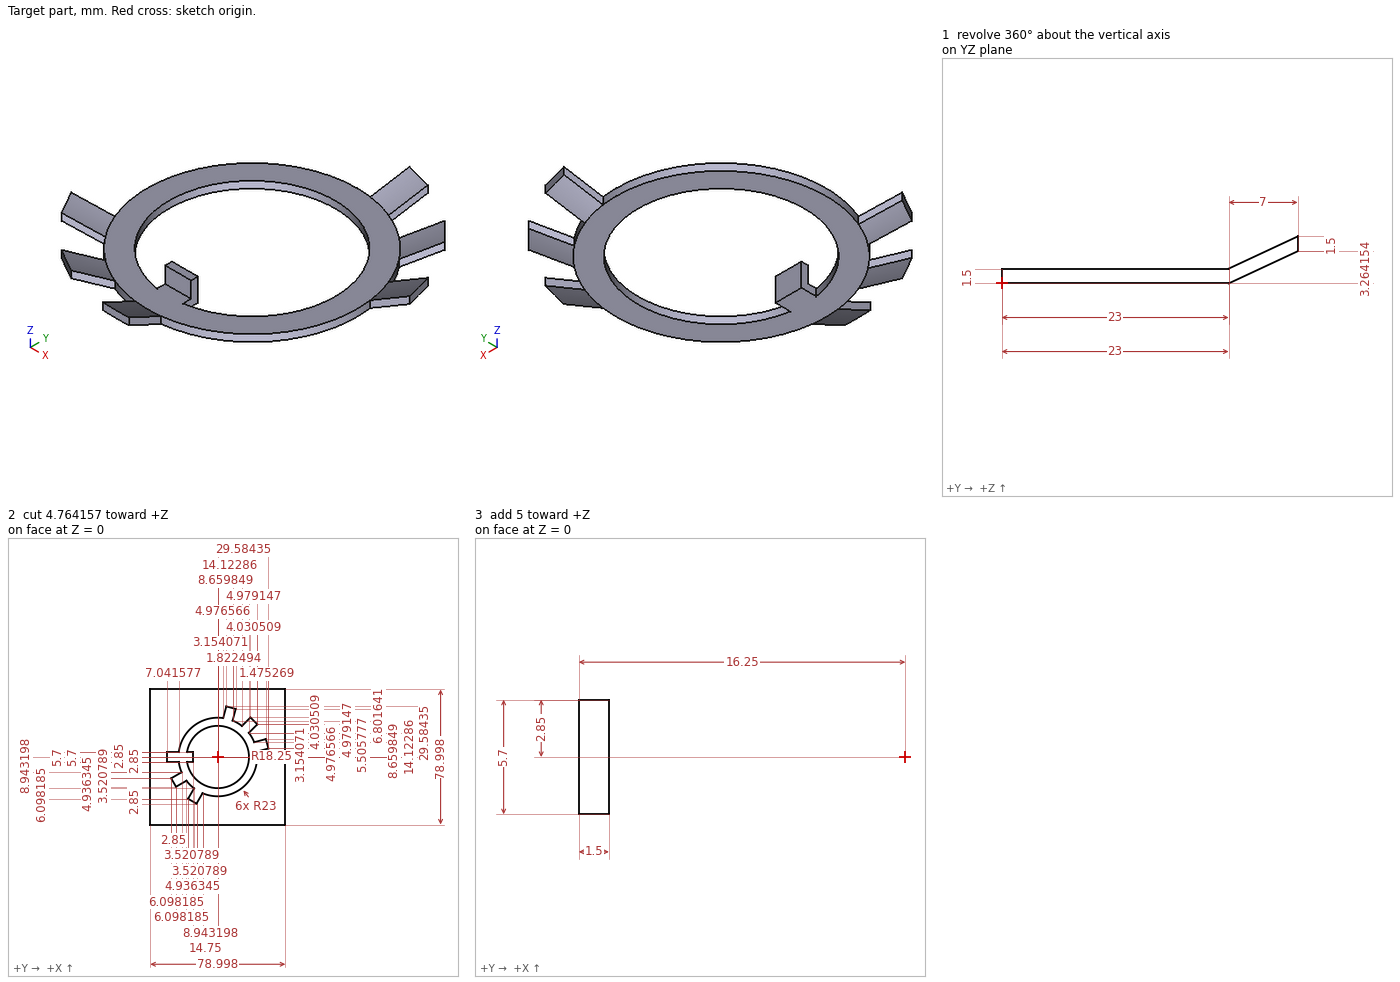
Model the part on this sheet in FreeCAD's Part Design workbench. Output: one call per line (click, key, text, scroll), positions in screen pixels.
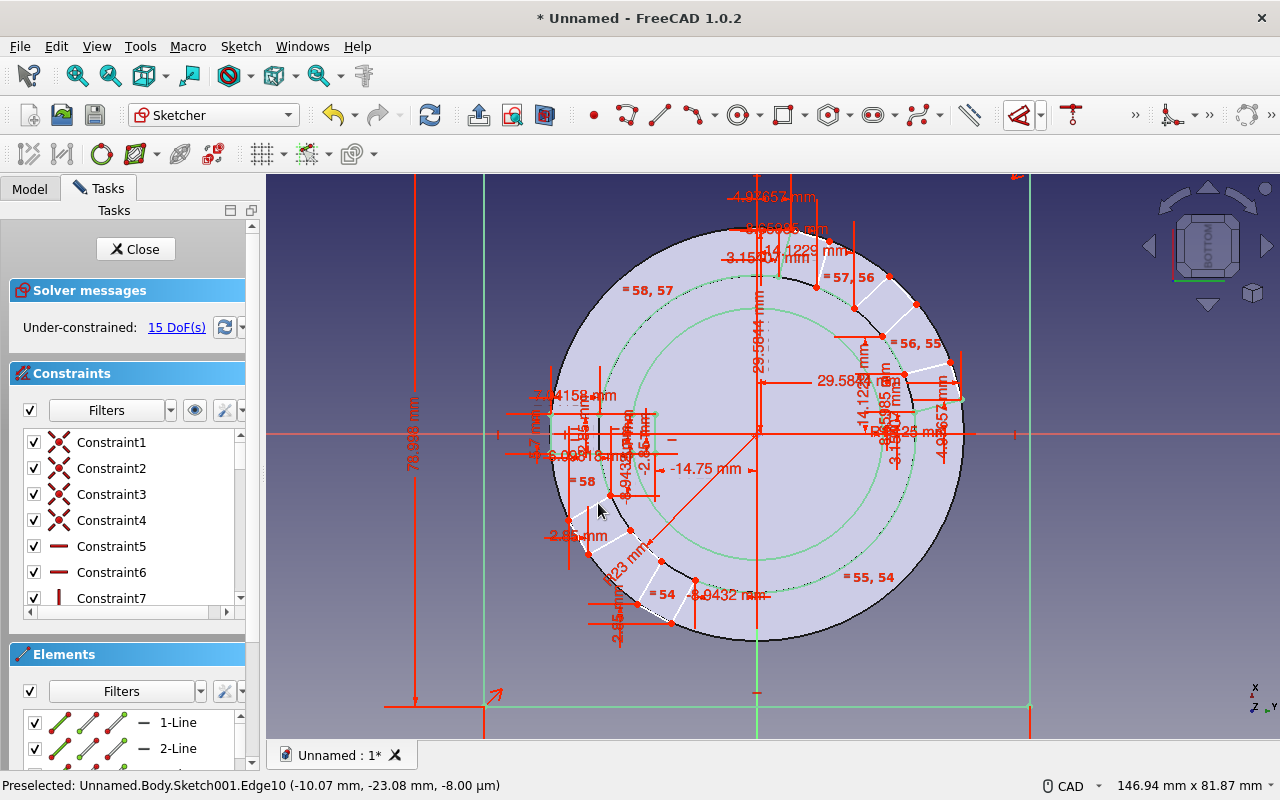
scroll(598, 503, up, 3)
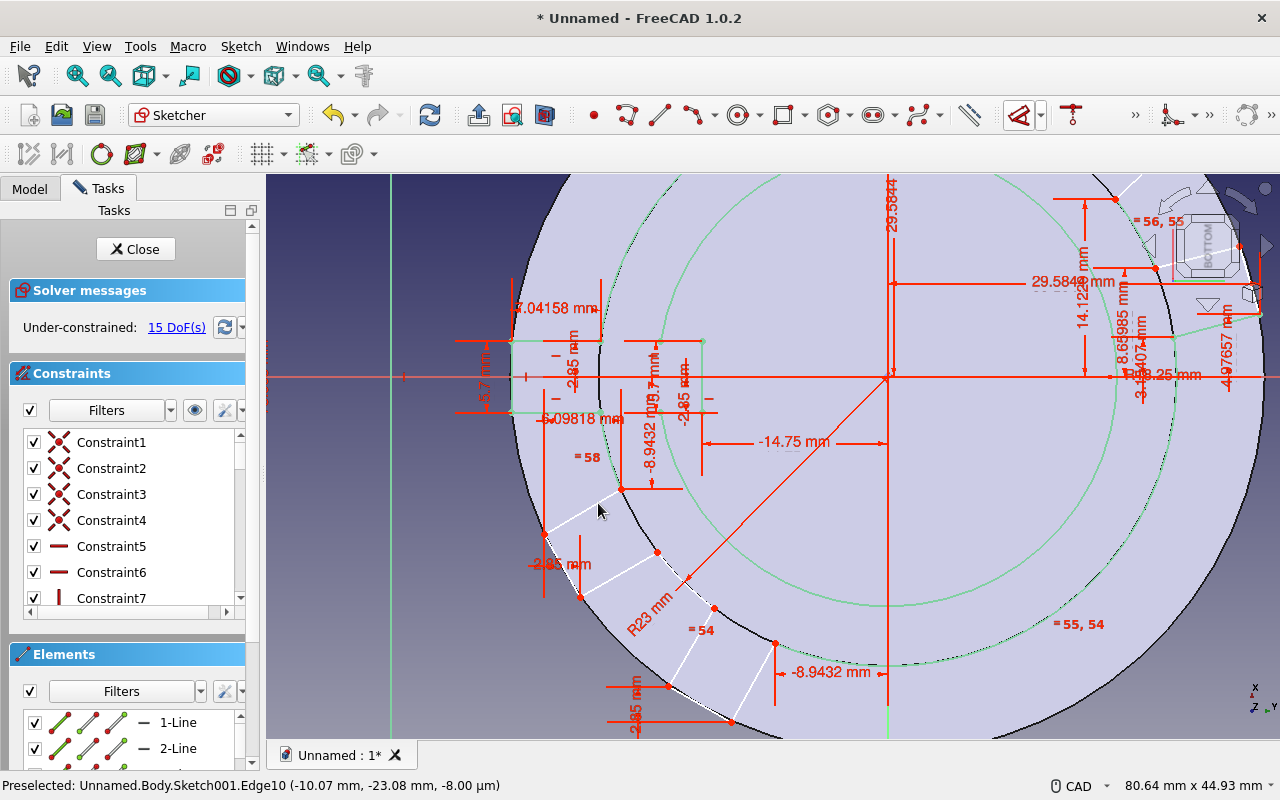
click(598, 503)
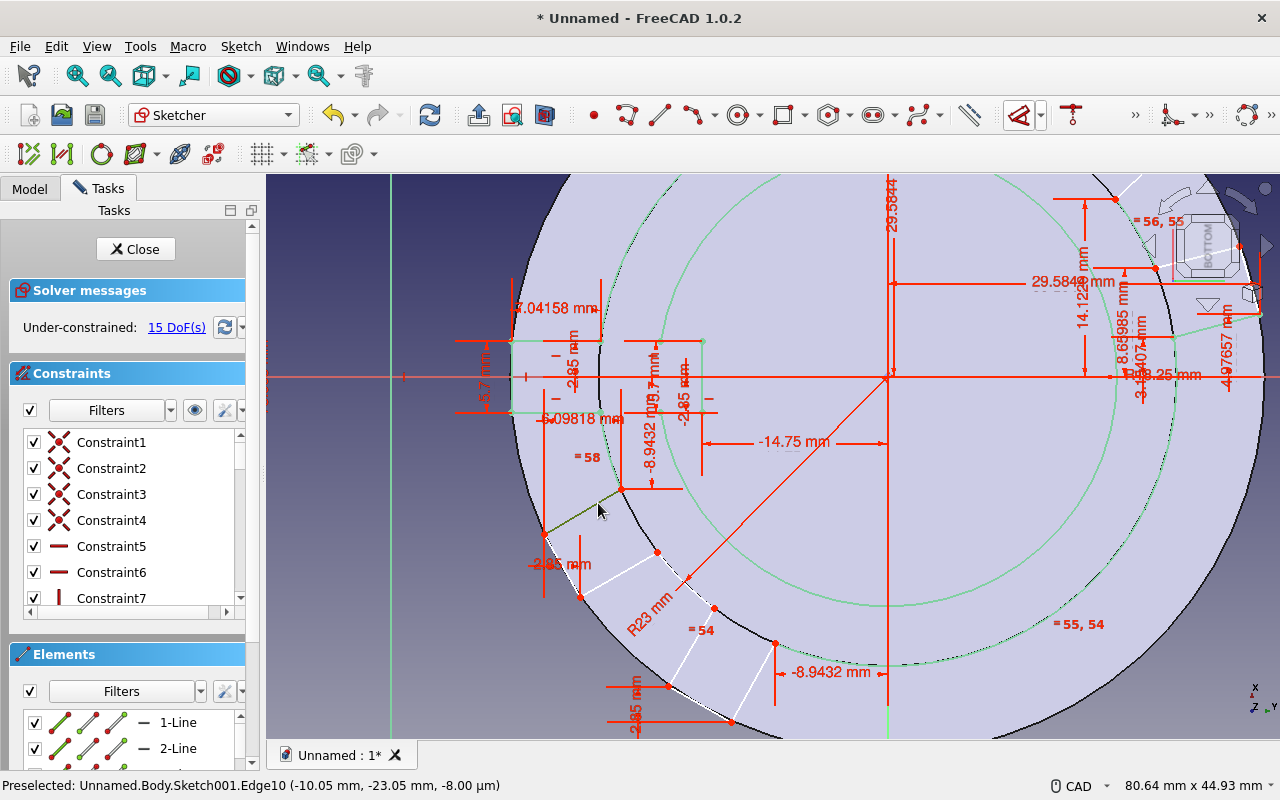
key(i)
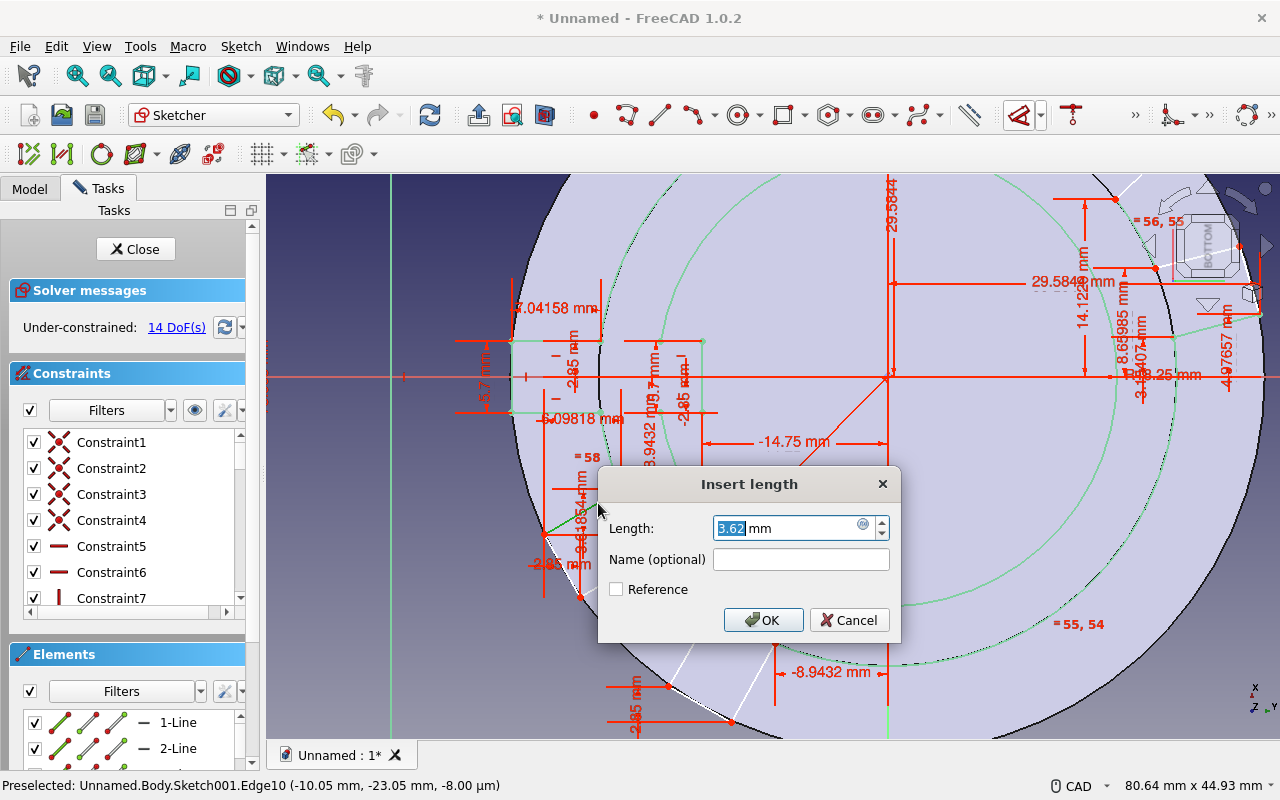
text(3.520789)
key(Return)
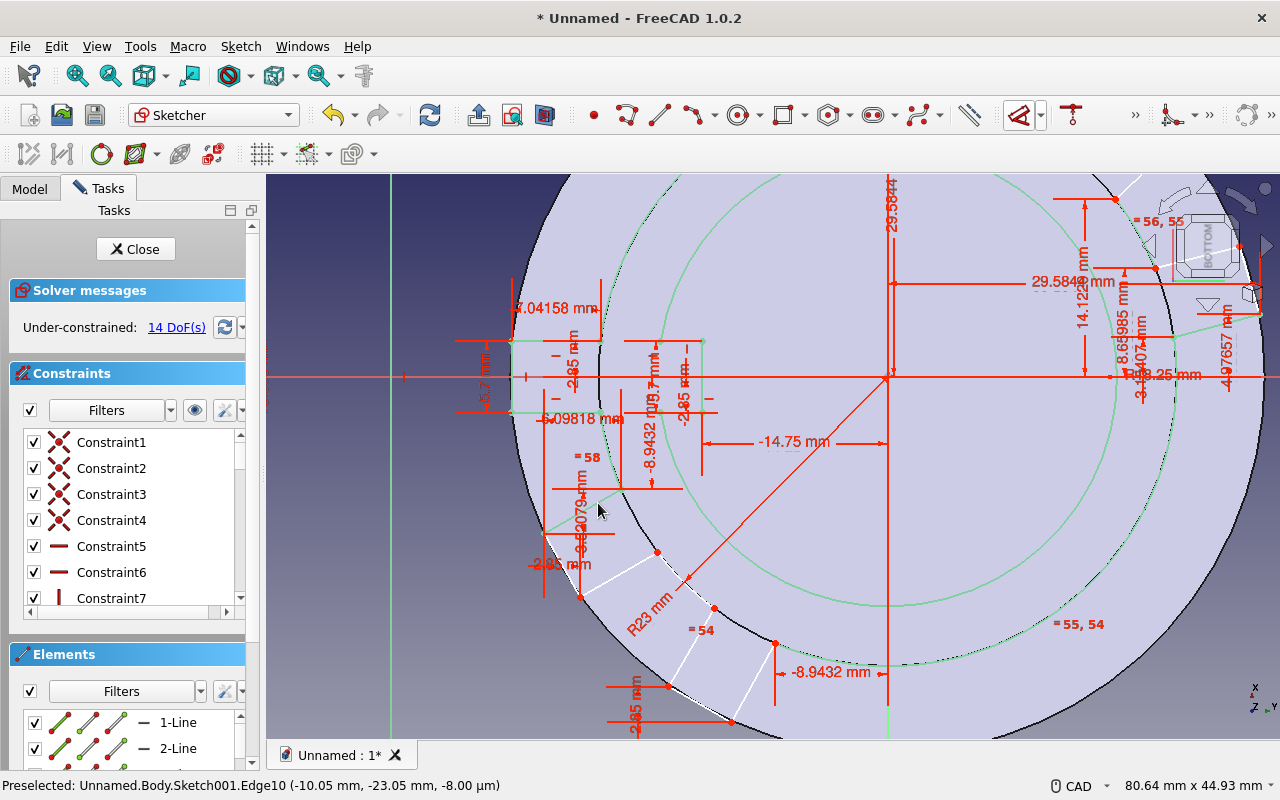
click(555, 553)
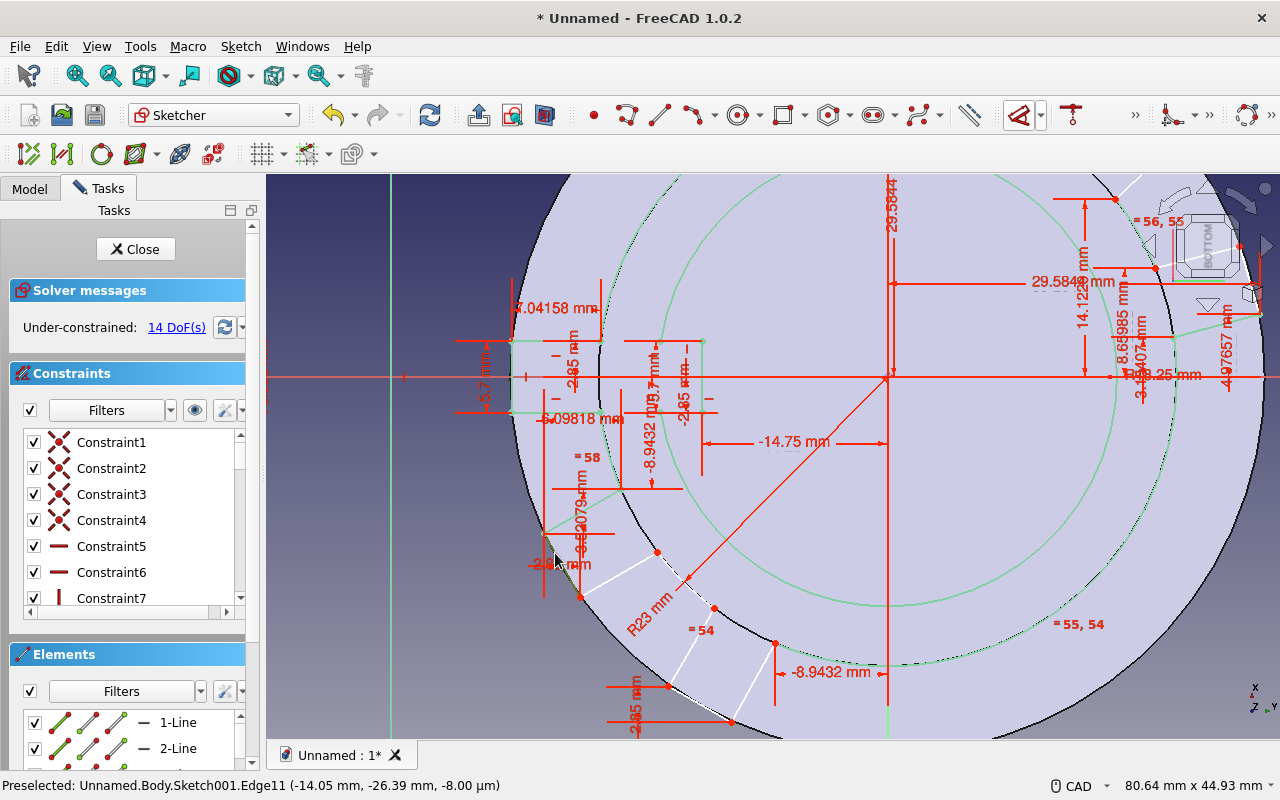
click(1040, 116)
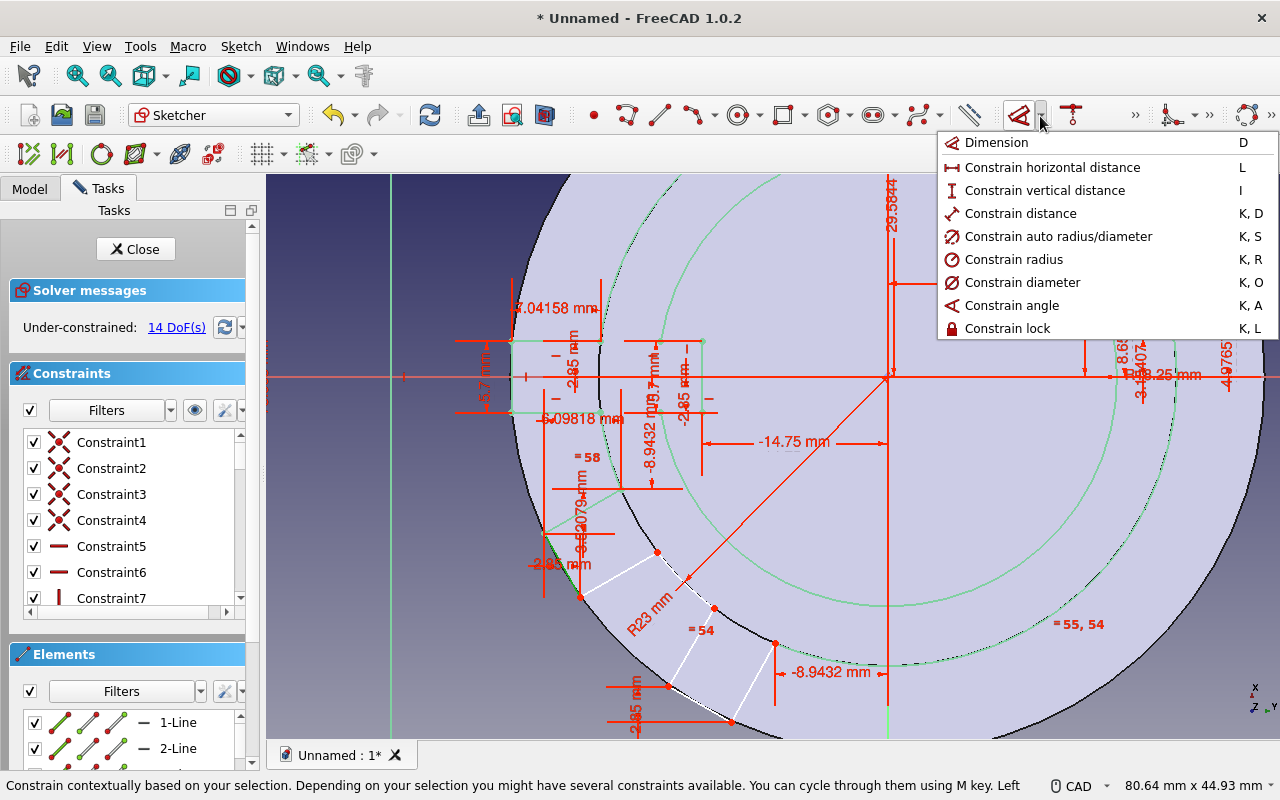
click(1108, 190)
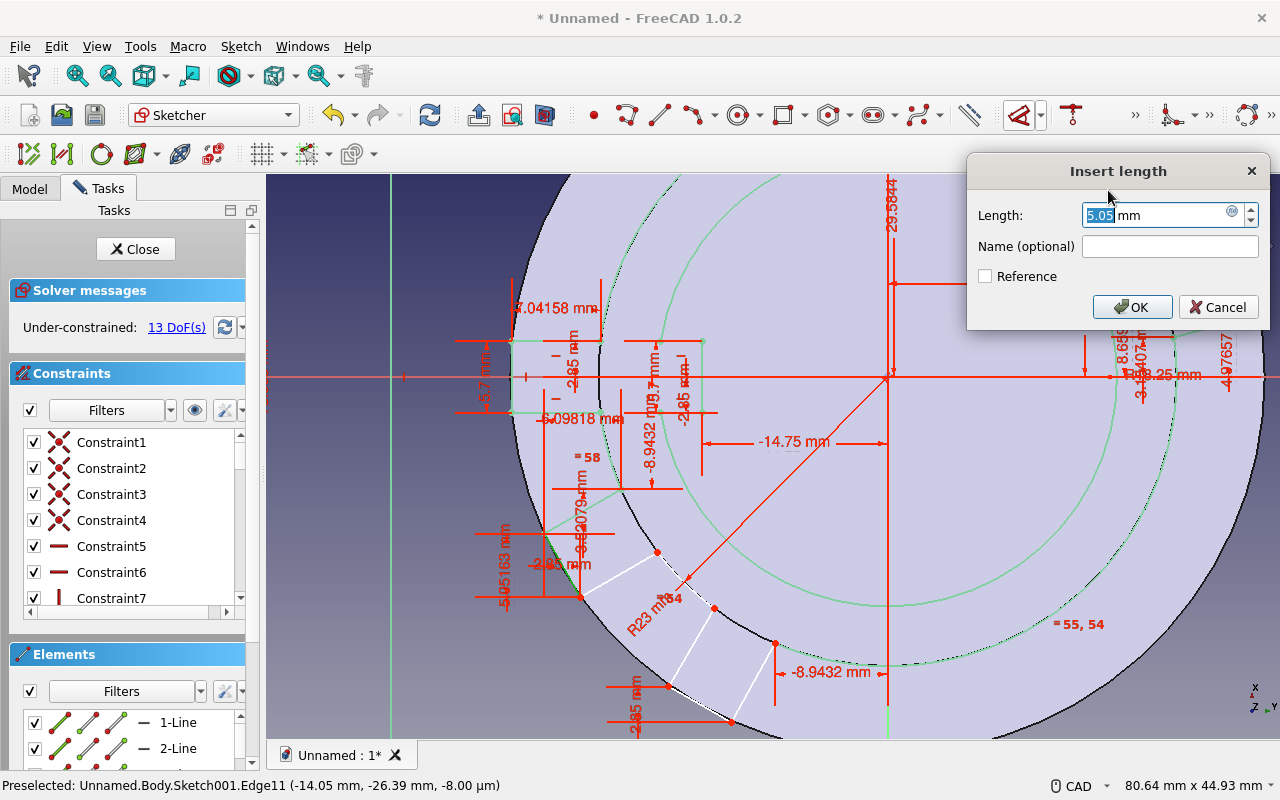
text(4.936345)
key(Return)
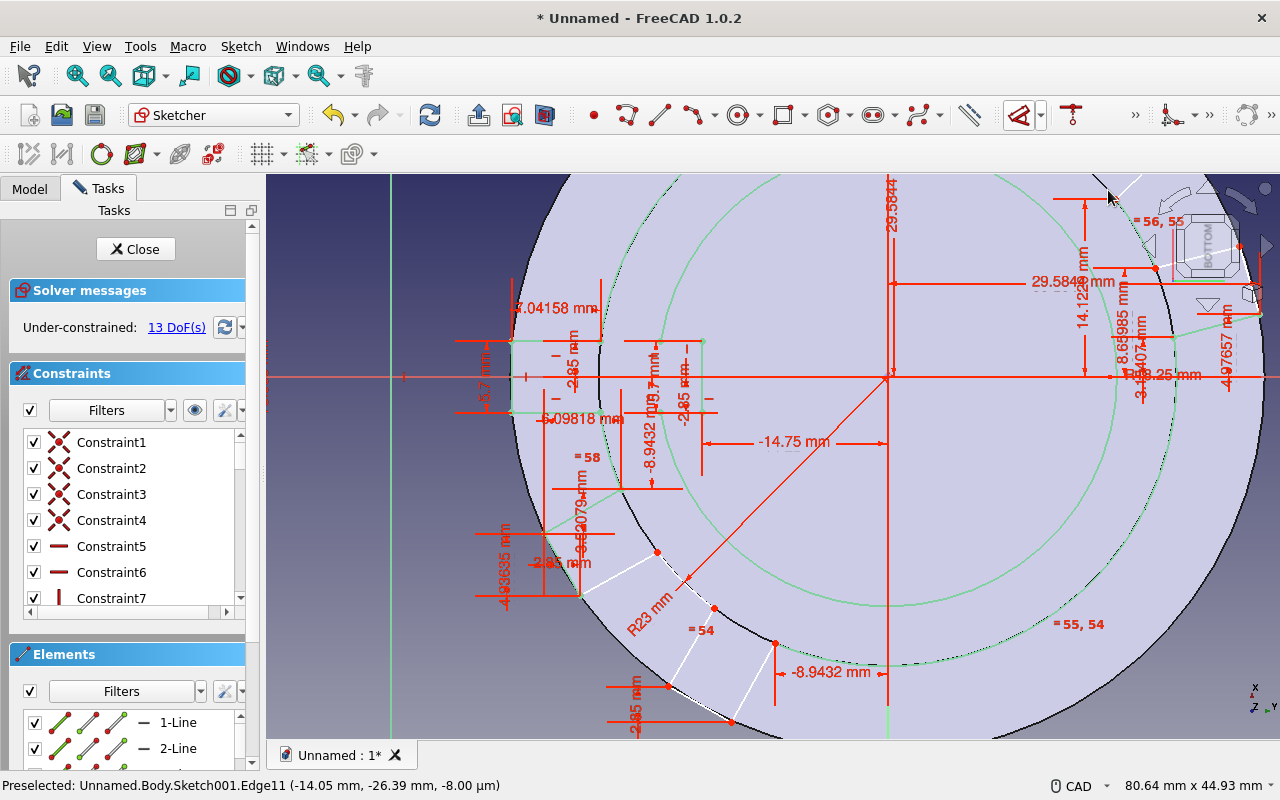
click(603, 583)